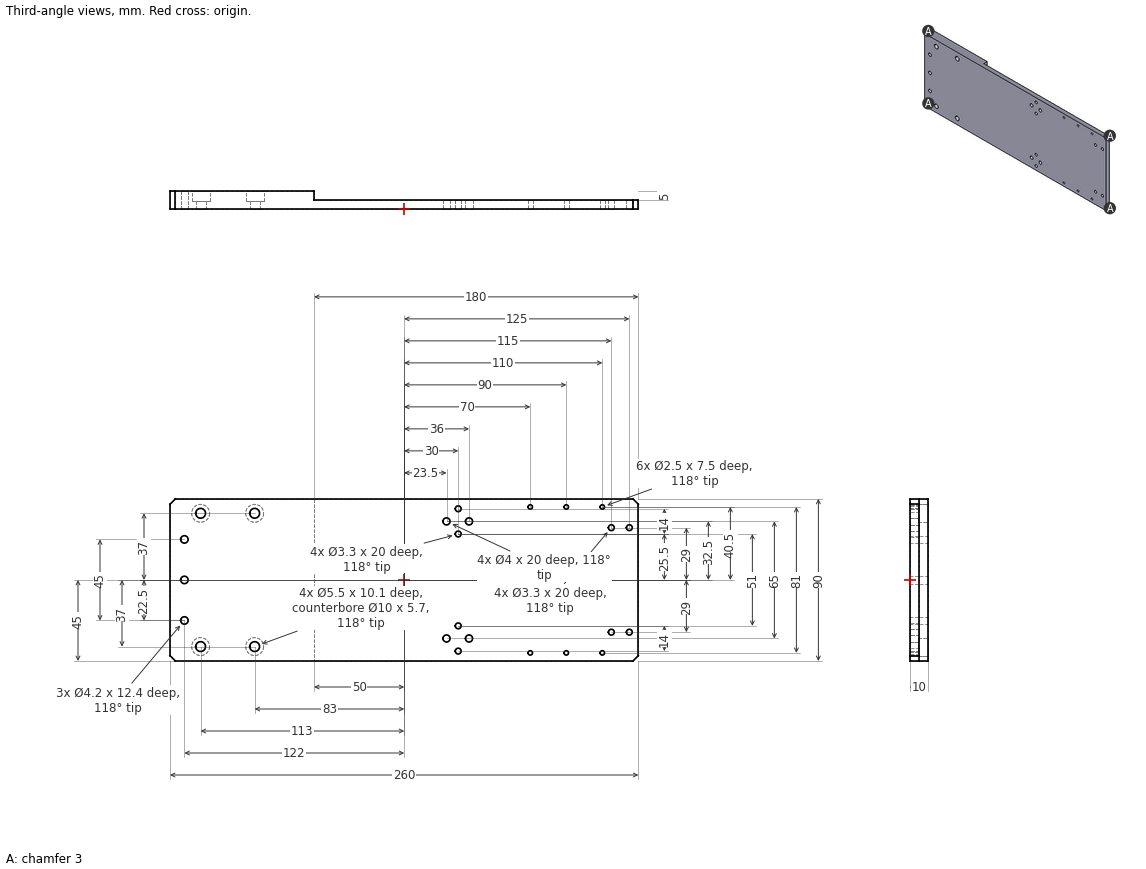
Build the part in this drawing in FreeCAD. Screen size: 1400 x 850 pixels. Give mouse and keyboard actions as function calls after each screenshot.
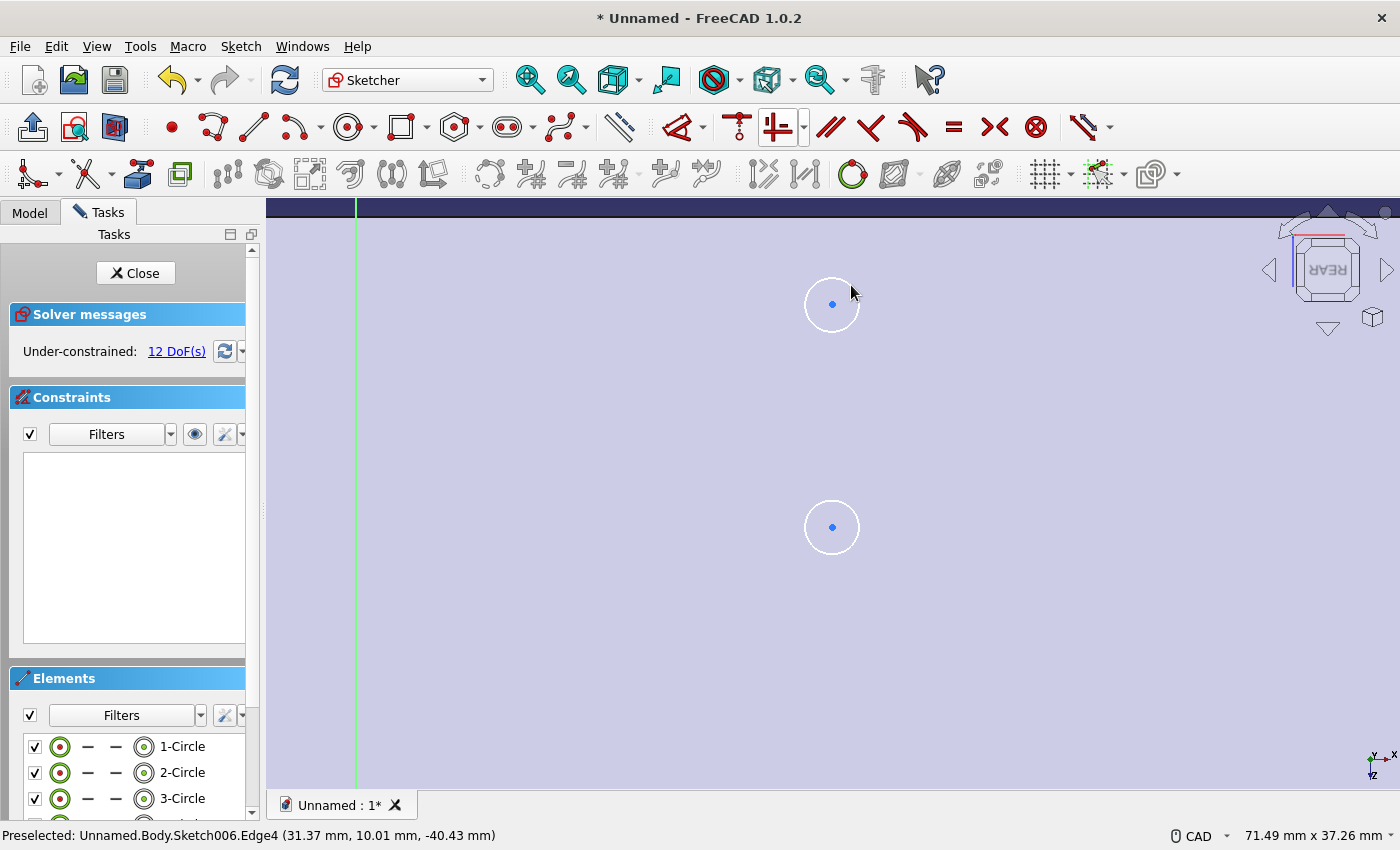
scroll(832, 305, down, 6)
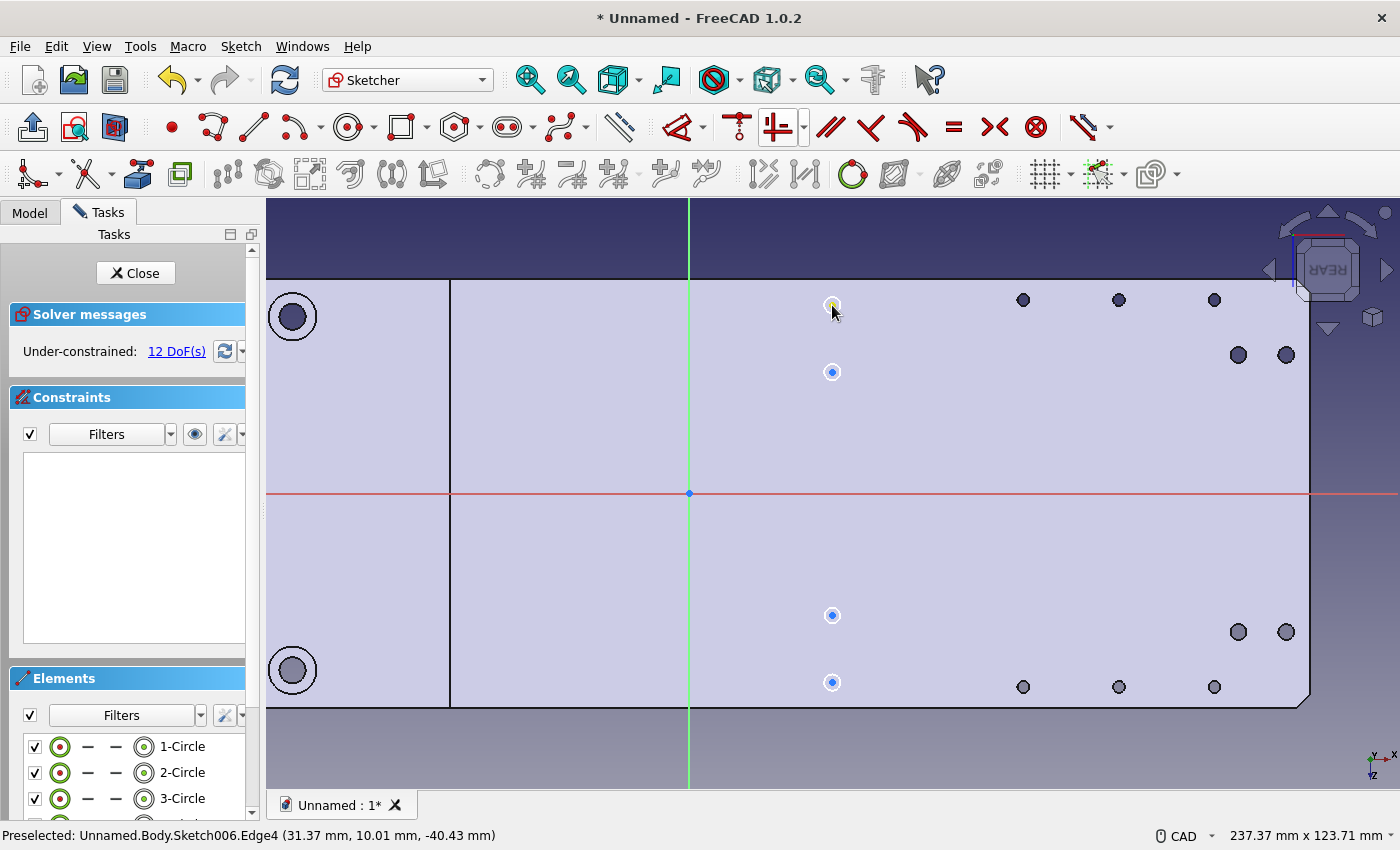
scroll(838, 610, up, 3)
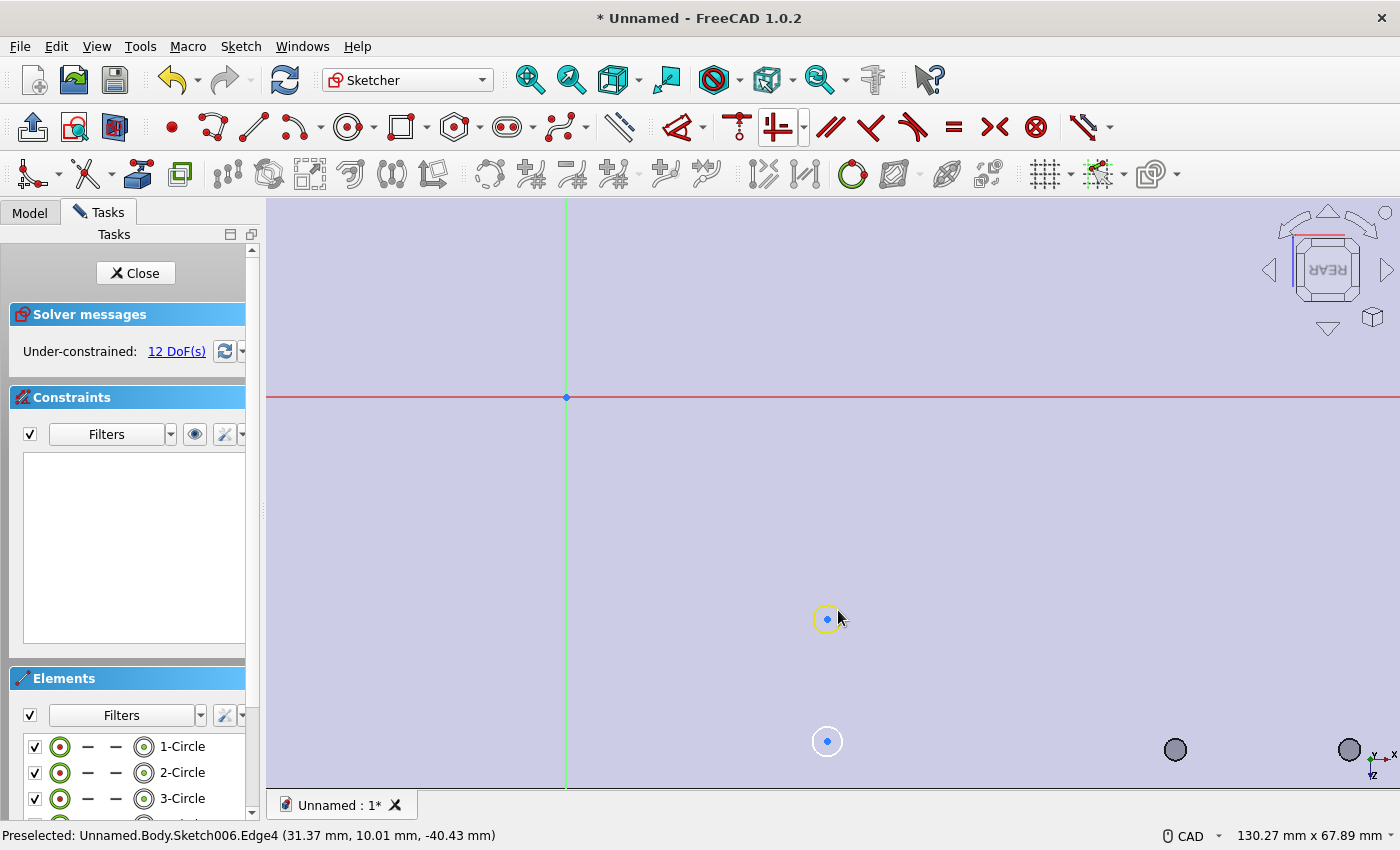
click(837, 610)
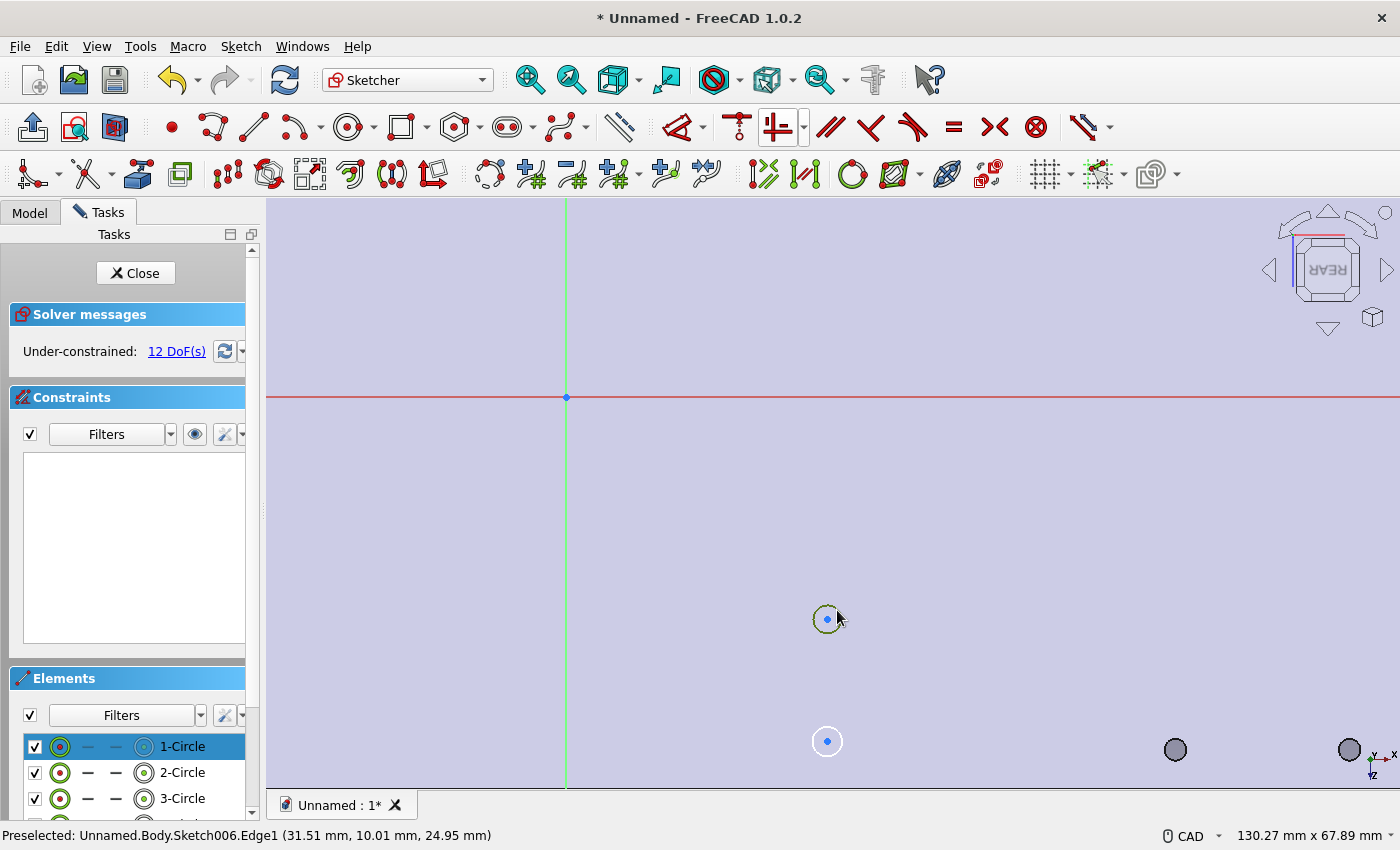
click(838, 731)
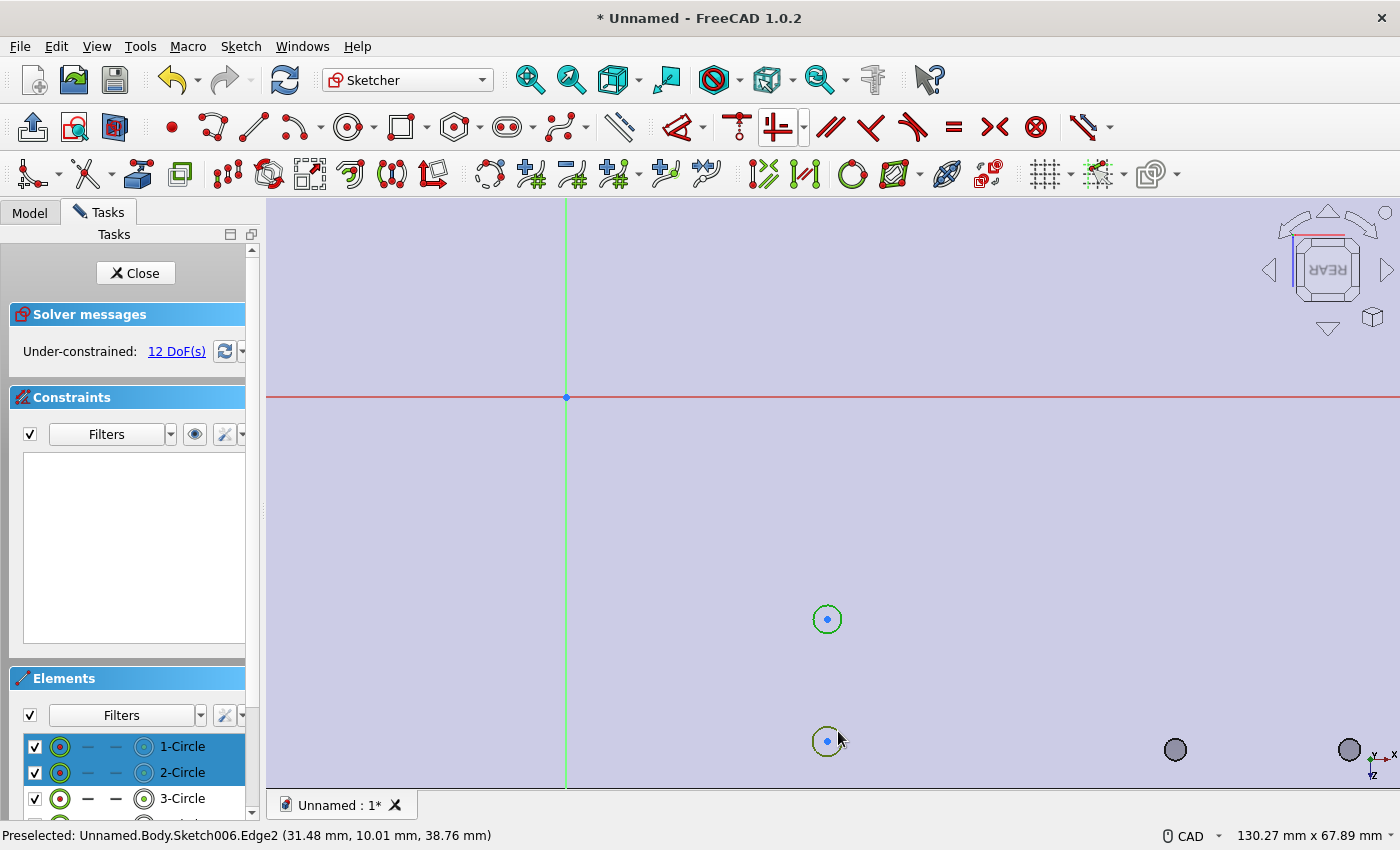
scroll(838, 611, down, 3)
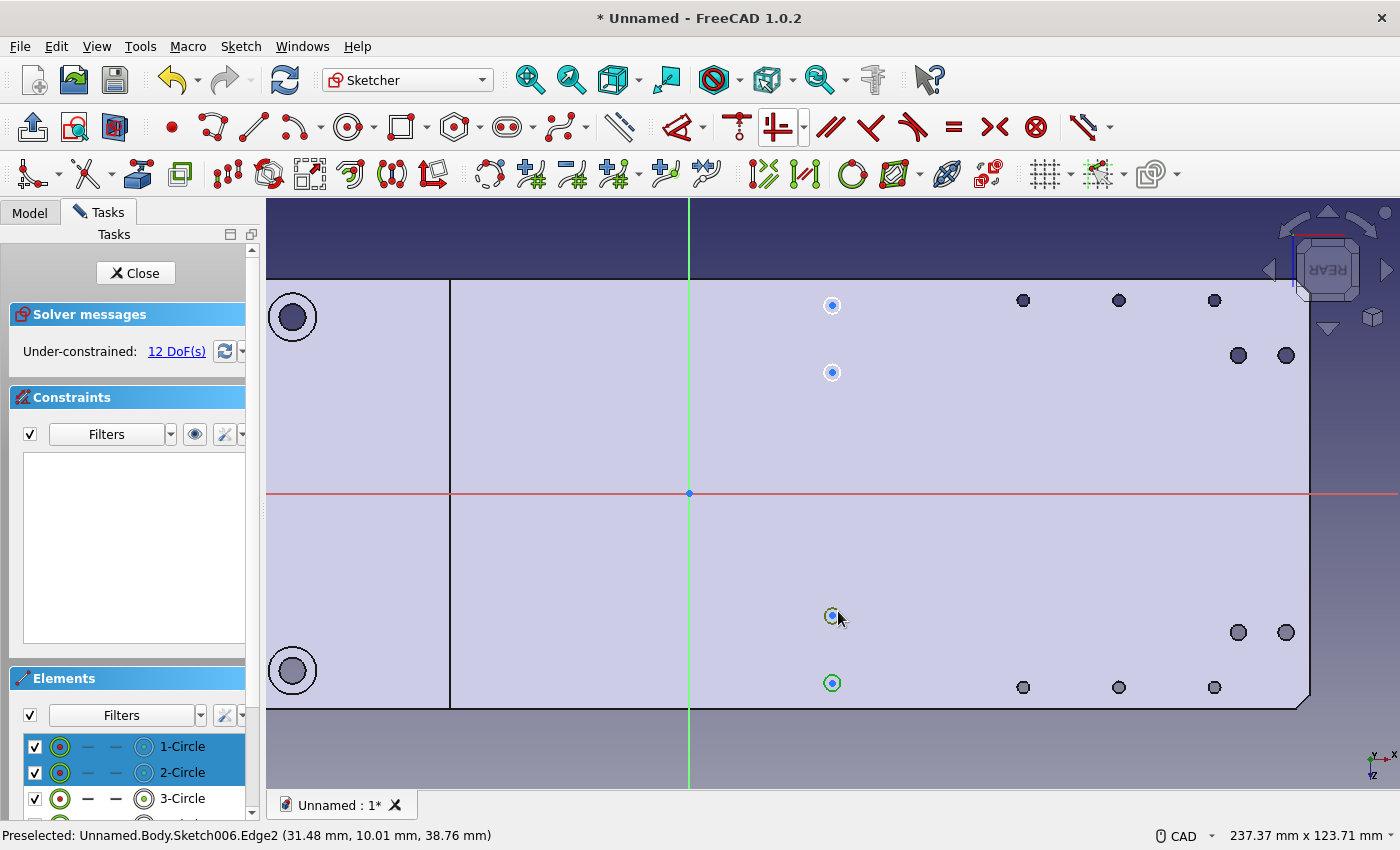
scroll(838, 367, up, 3)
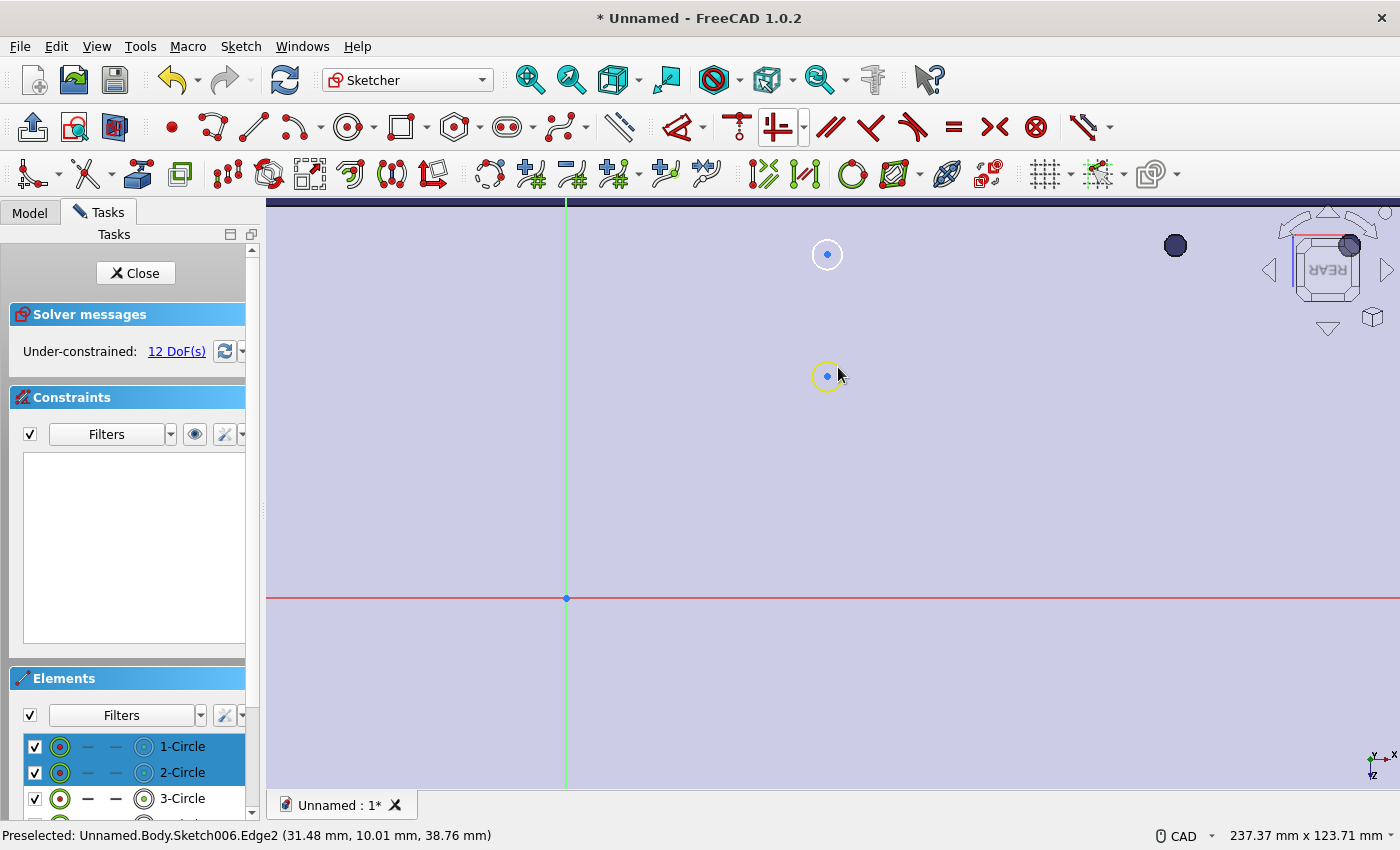
click(838, 366)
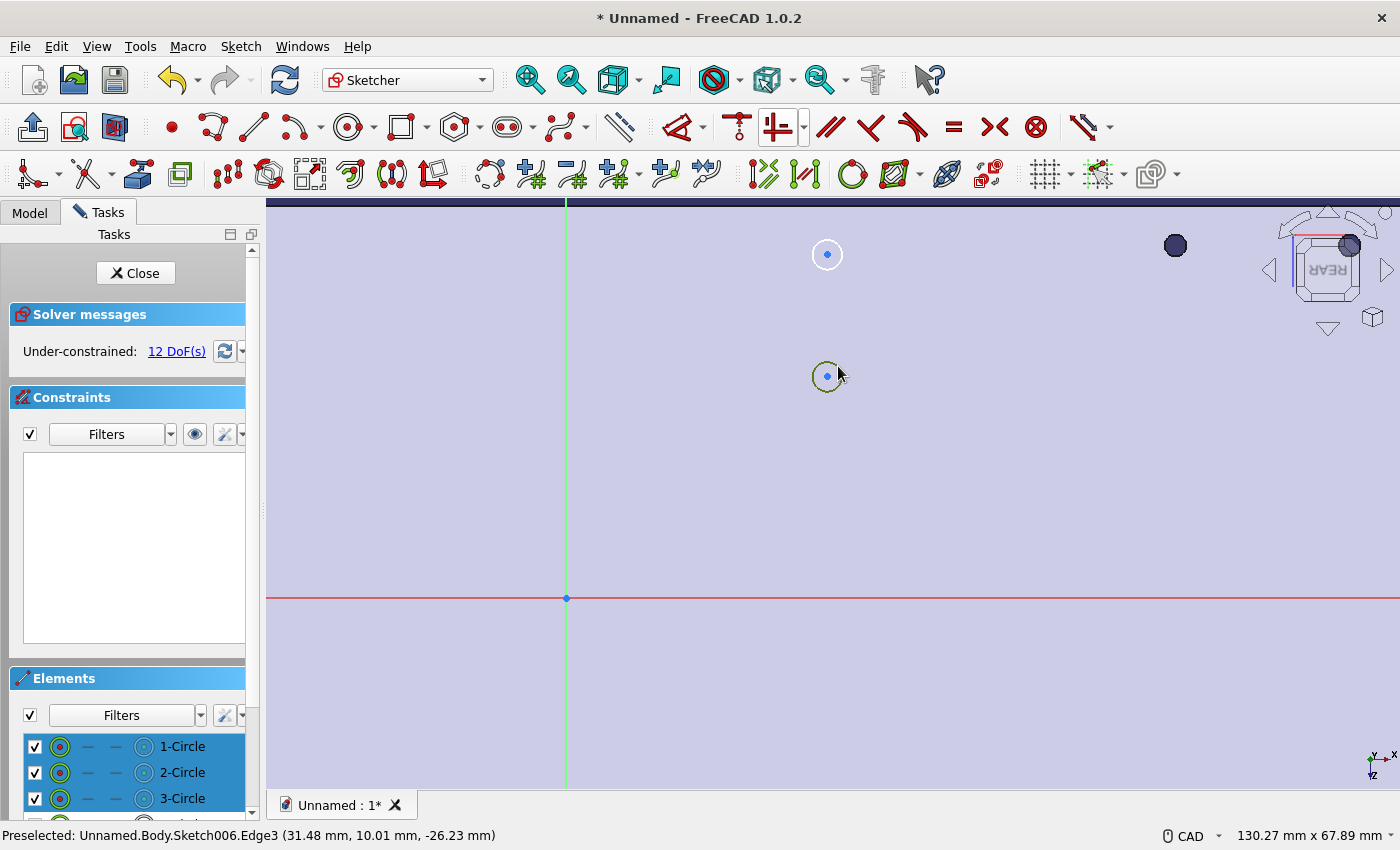
click(838, 244)